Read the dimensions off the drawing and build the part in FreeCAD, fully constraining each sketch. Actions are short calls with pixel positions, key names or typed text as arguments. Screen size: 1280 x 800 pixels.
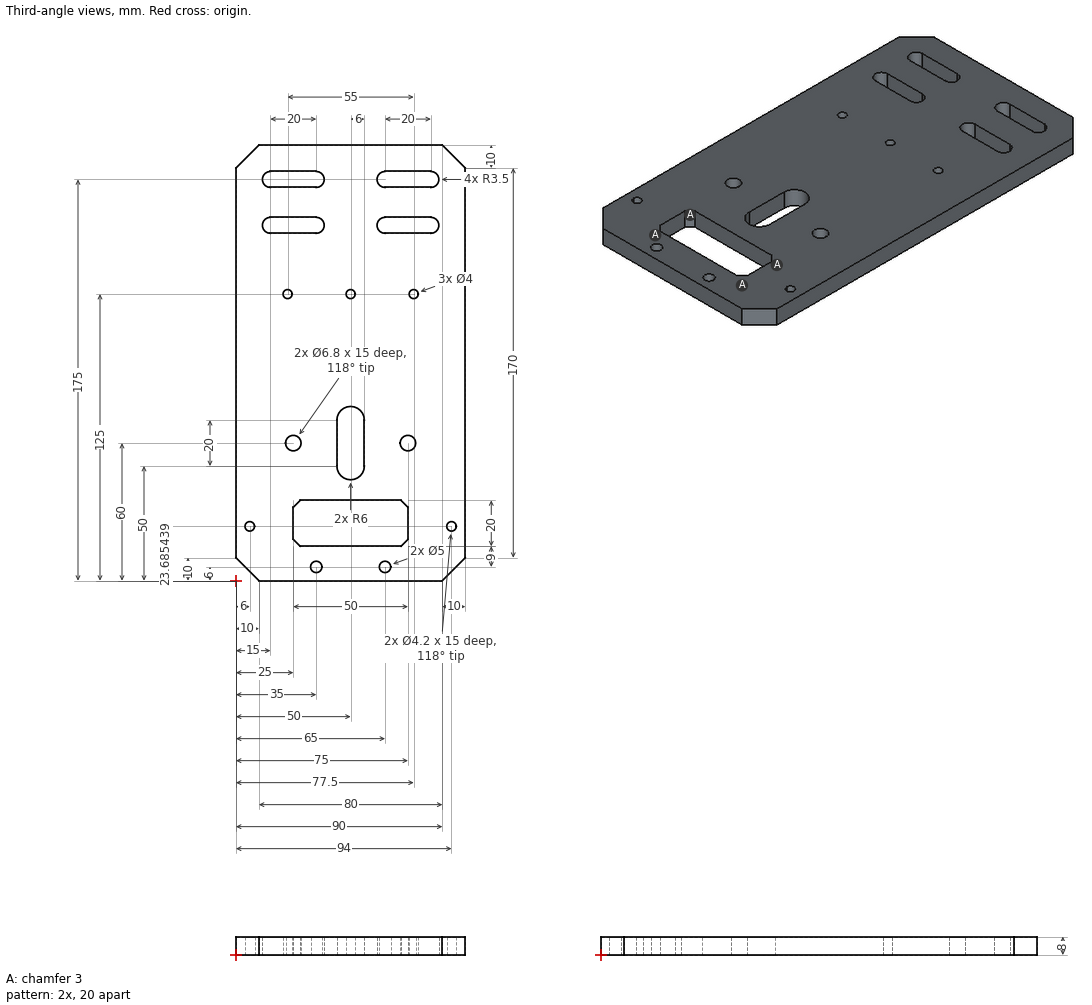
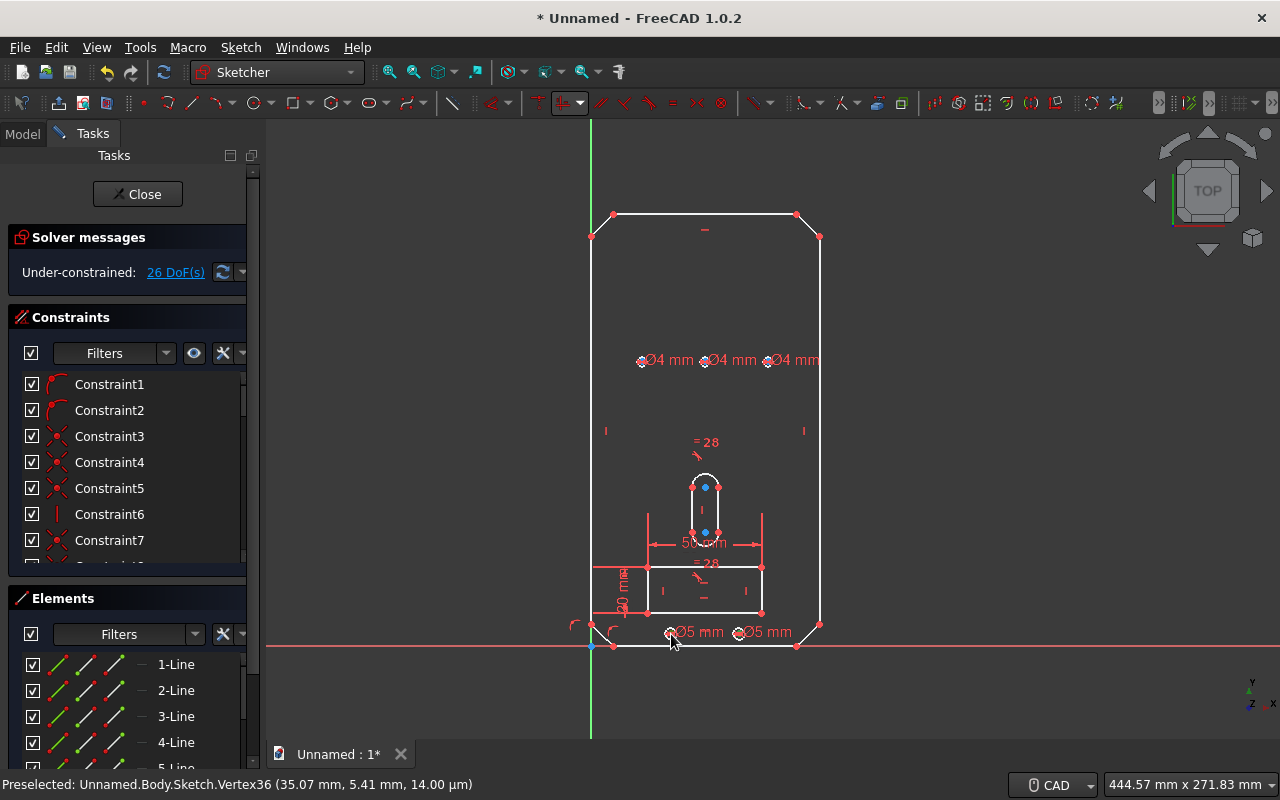
click(582, 104)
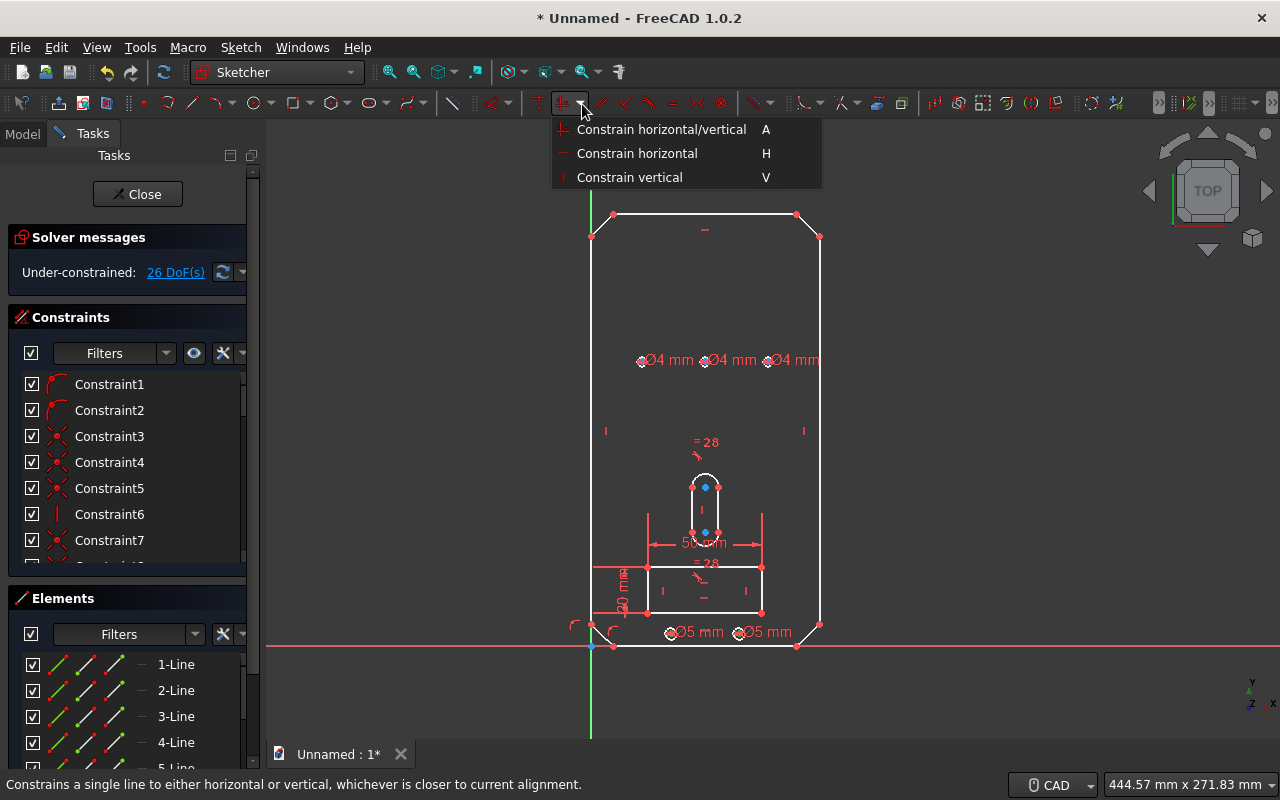
click(687, 153)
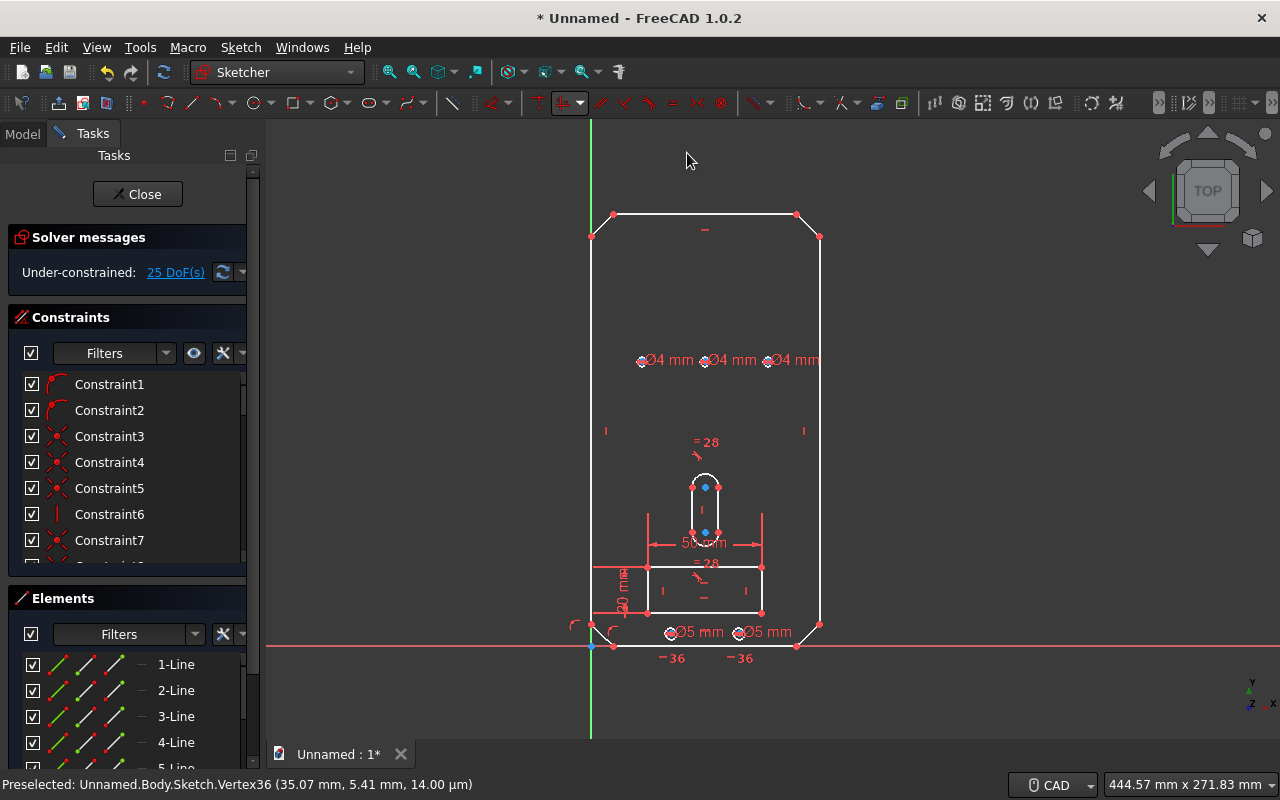
click(768, 362)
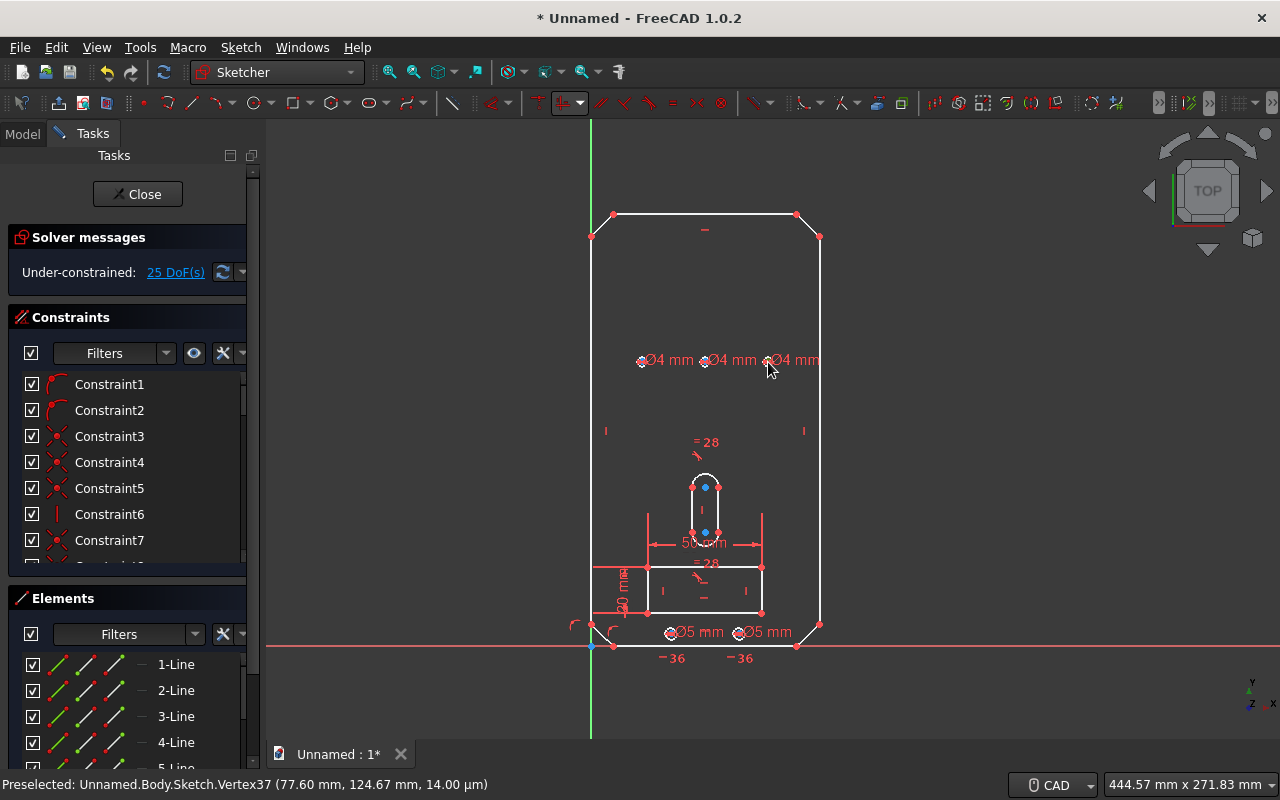
click(705, 362)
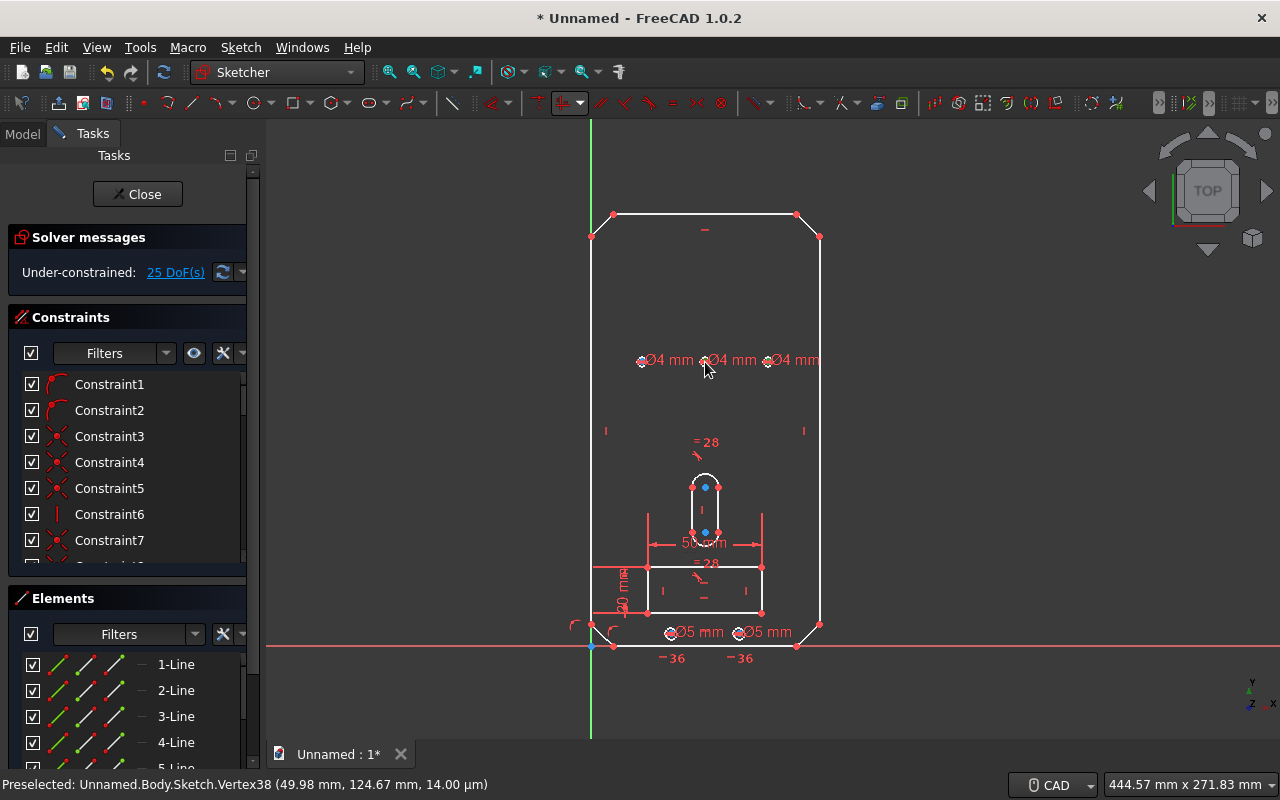
key(h)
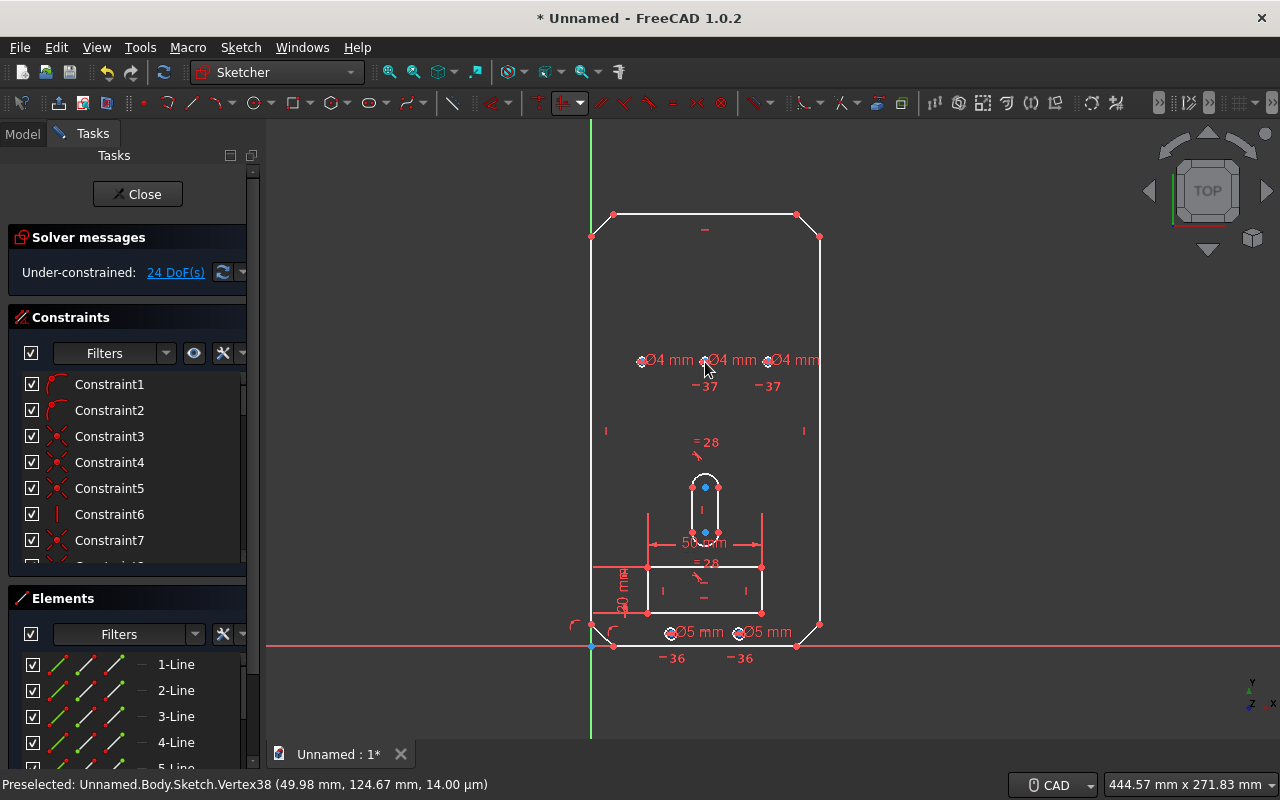
click(705, 362)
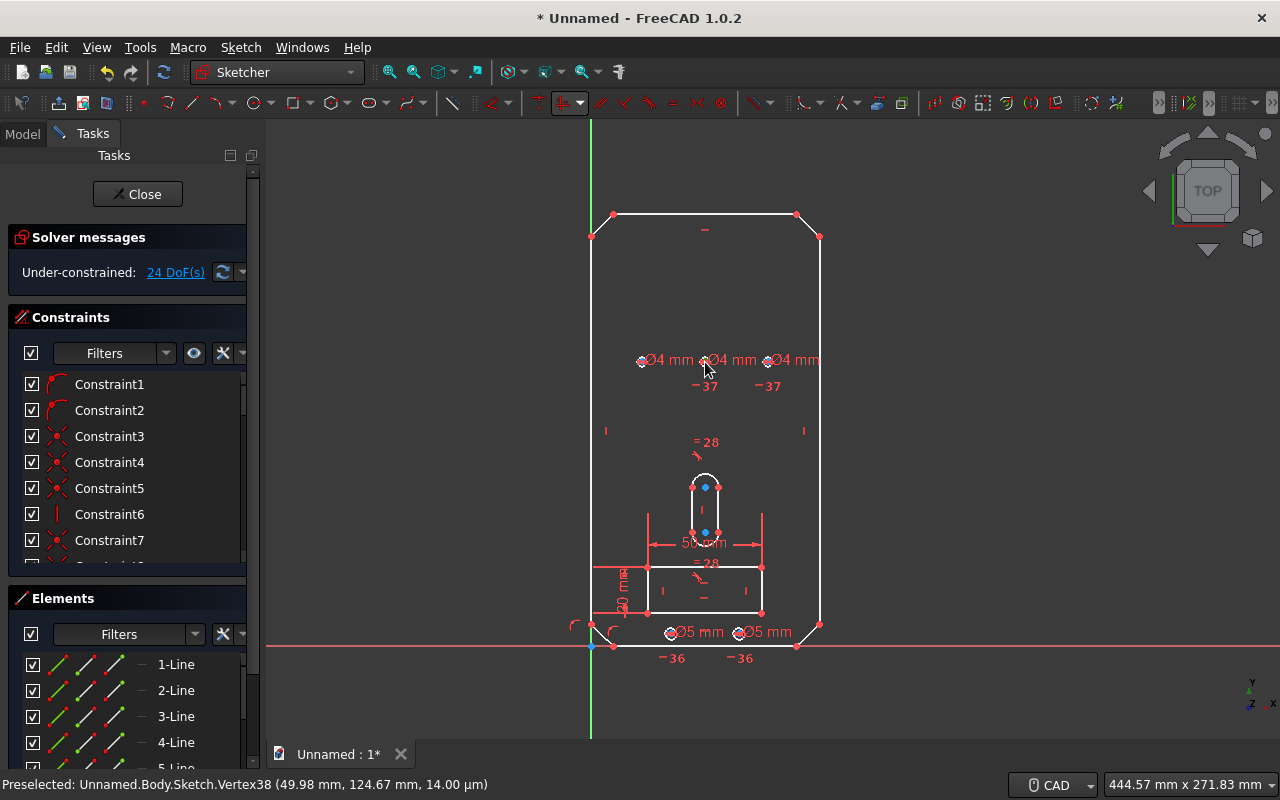
click(642, 362)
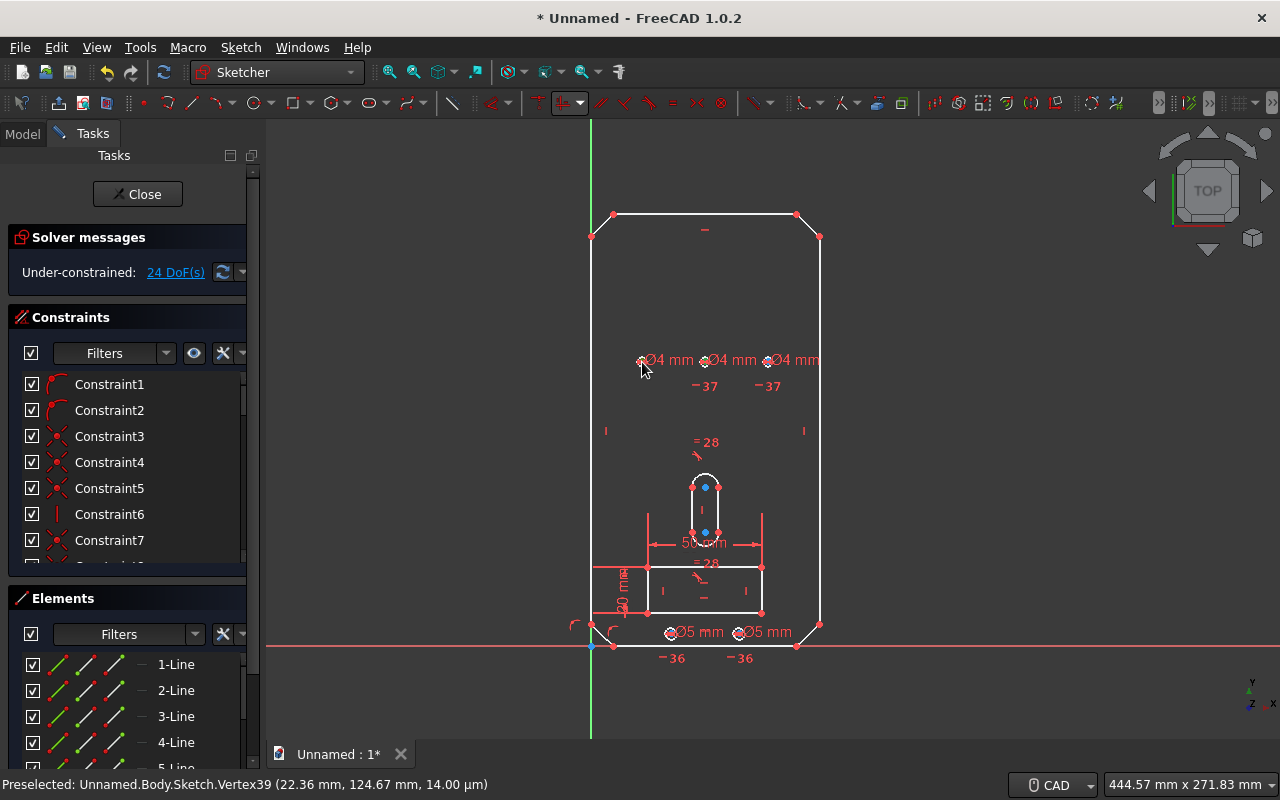
click(582, 104)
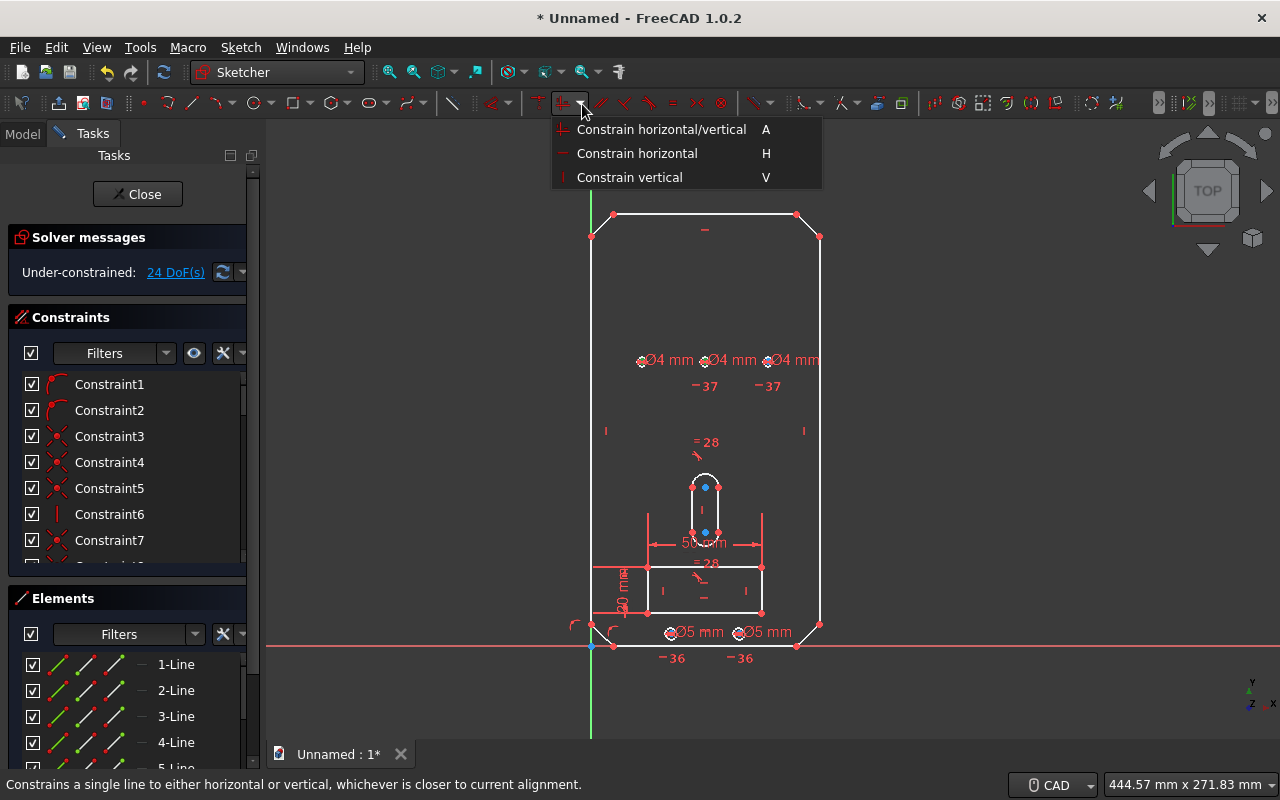
click(687, 153)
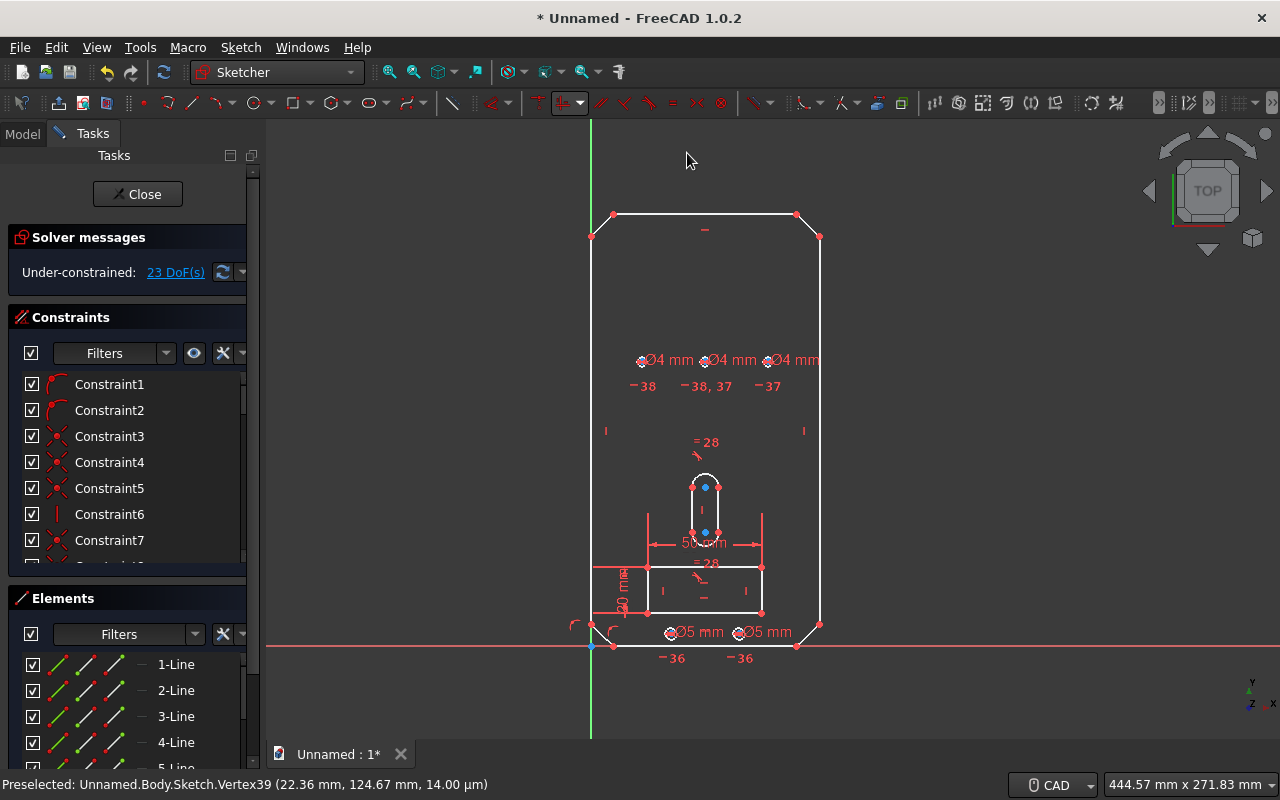
click(492, 104)